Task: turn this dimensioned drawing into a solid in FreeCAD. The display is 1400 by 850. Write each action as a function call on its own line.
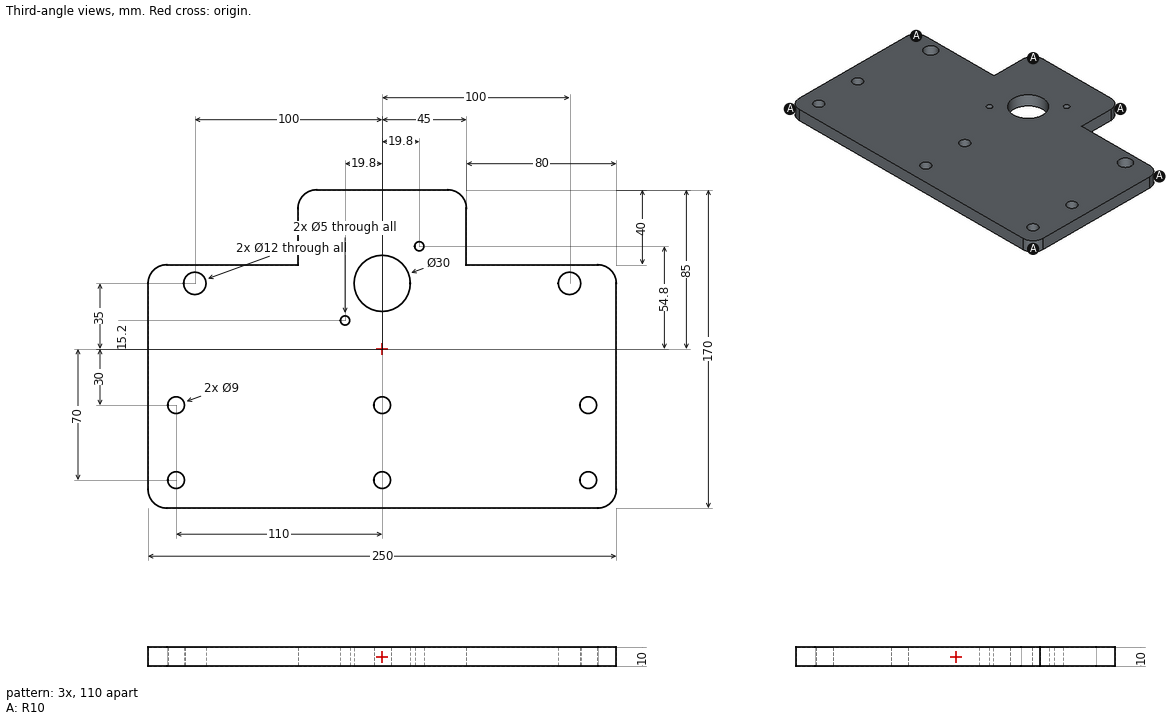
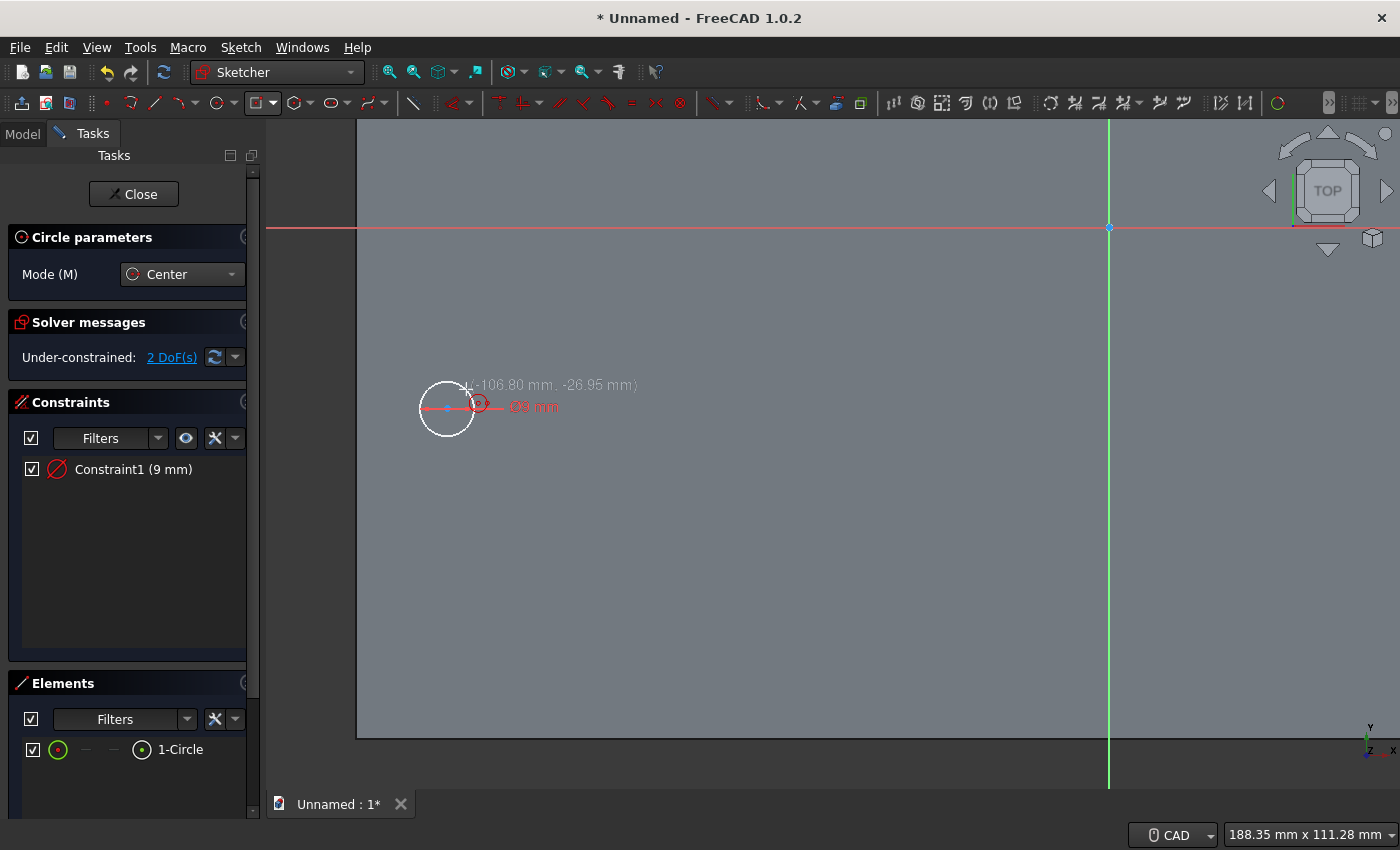
click(447, 649)
move(466, 630)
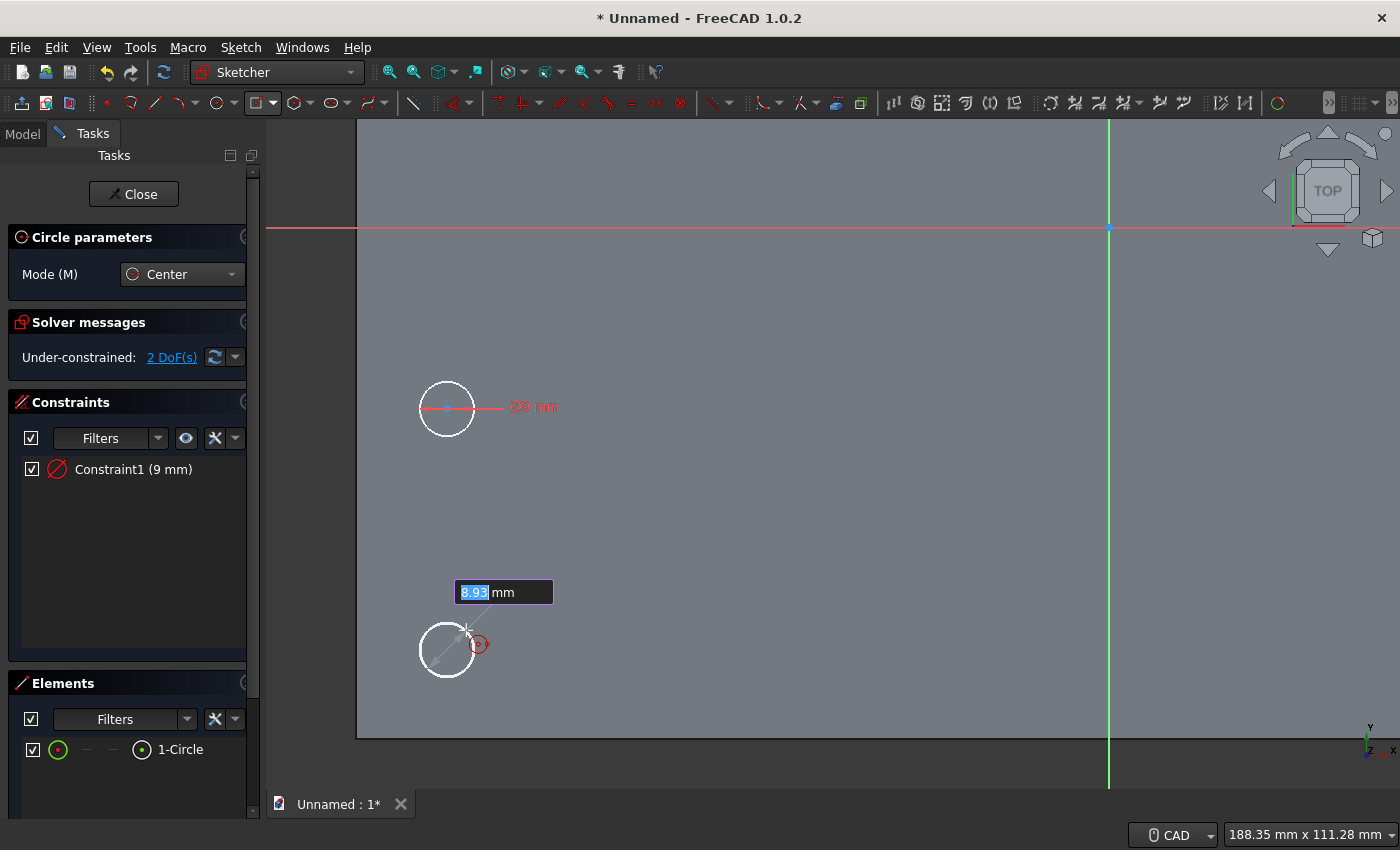
text(9)
key(Return)
key(Escape)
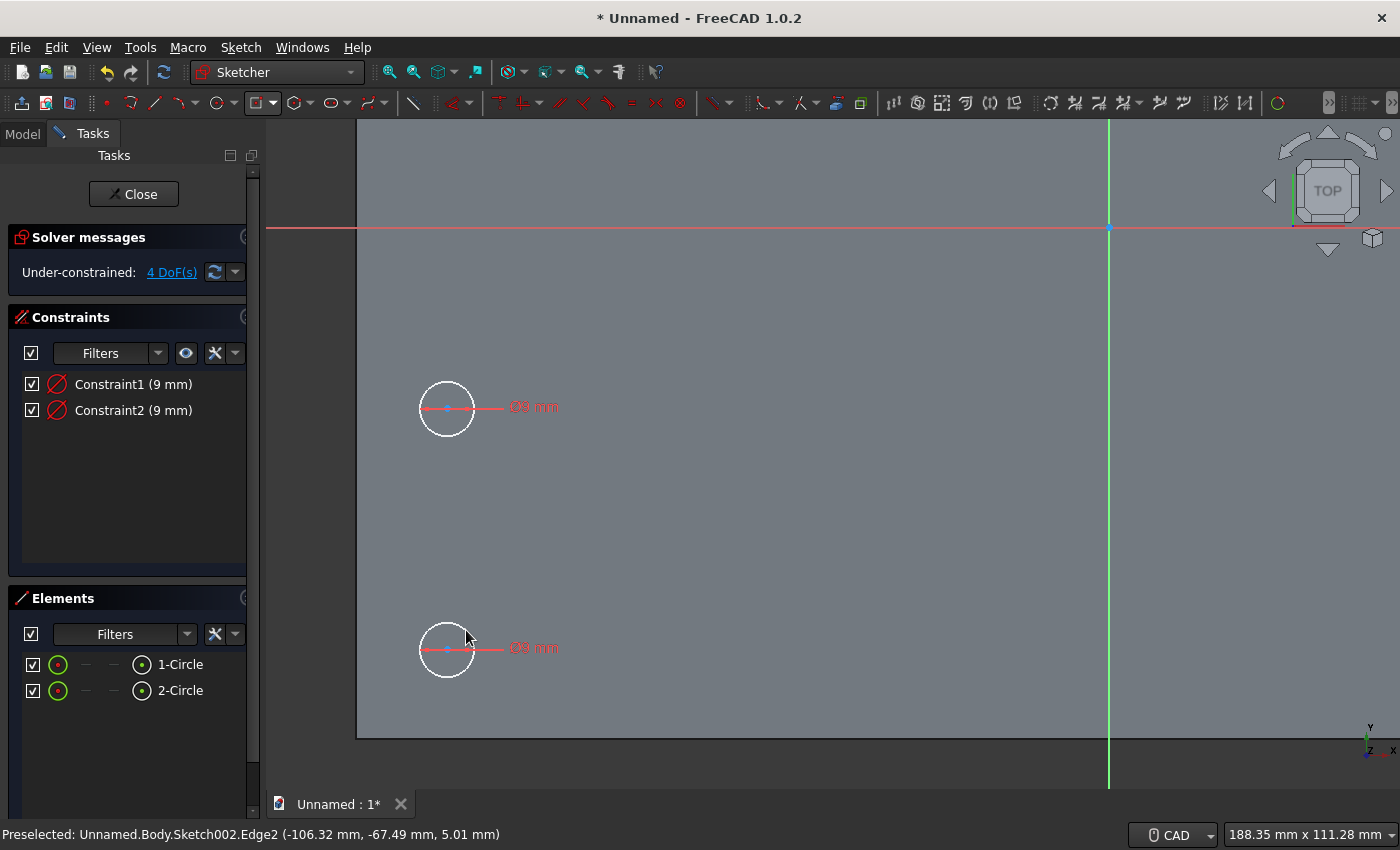
click(447, 409)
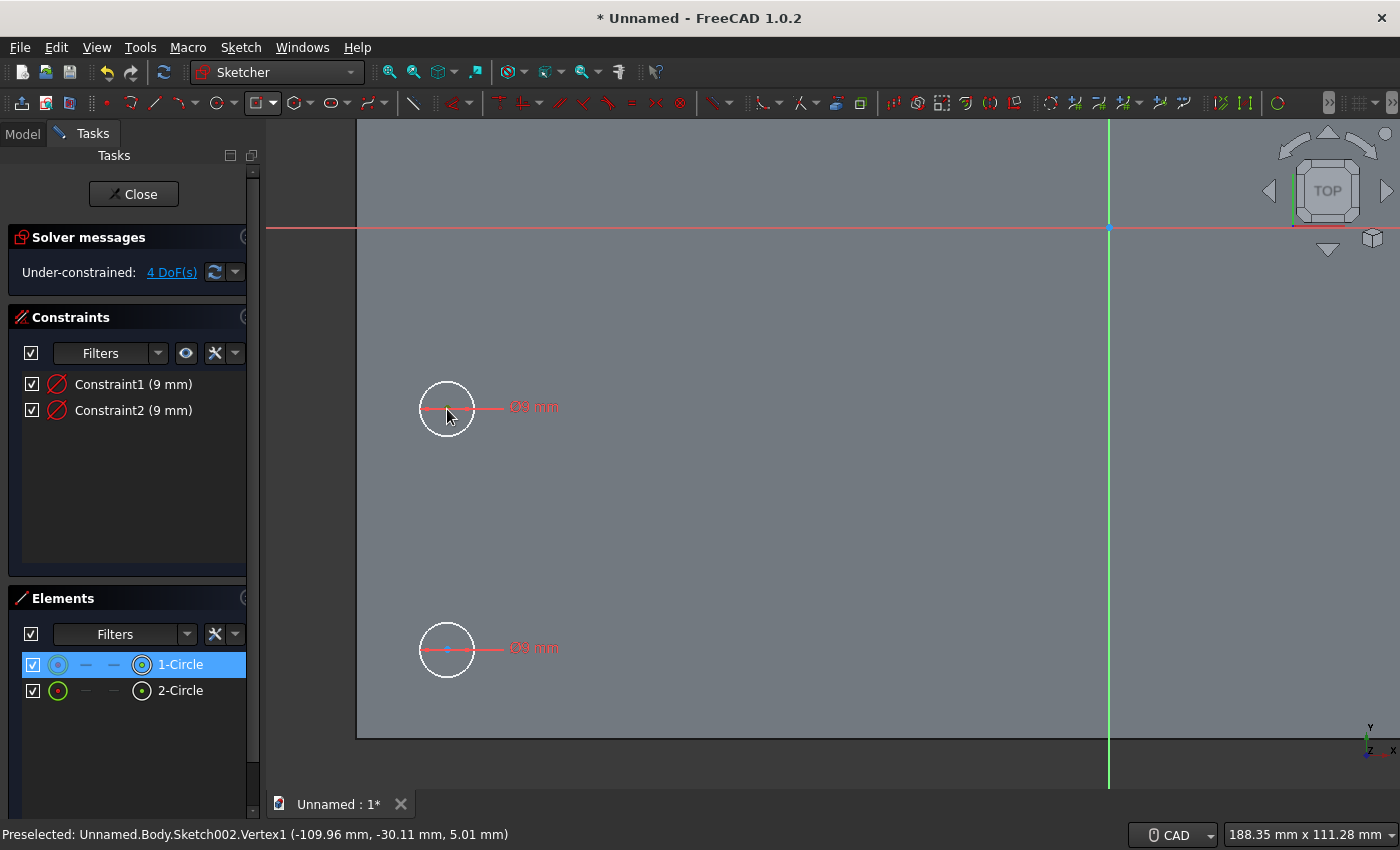
click(447, 650)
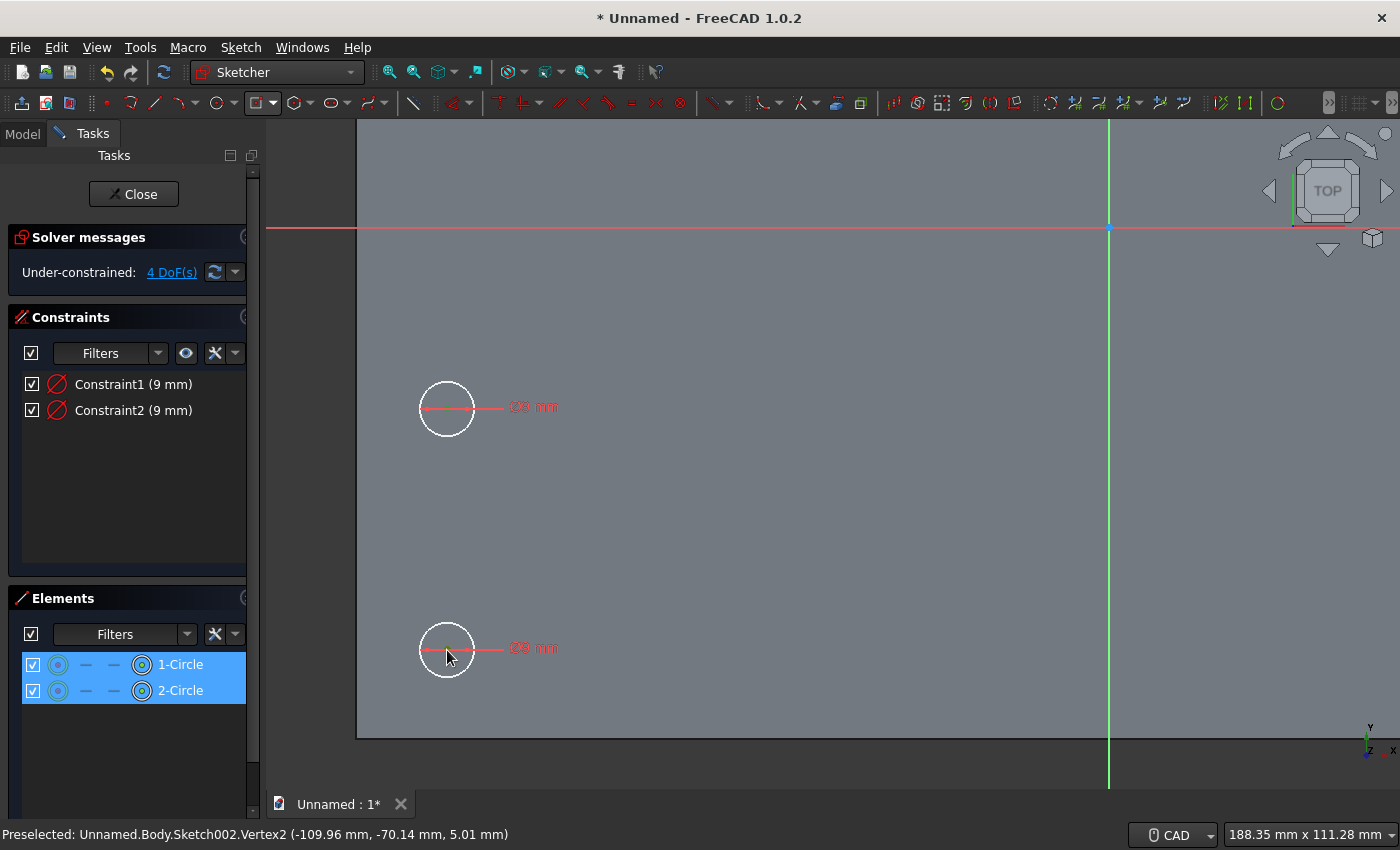
click(542, 104)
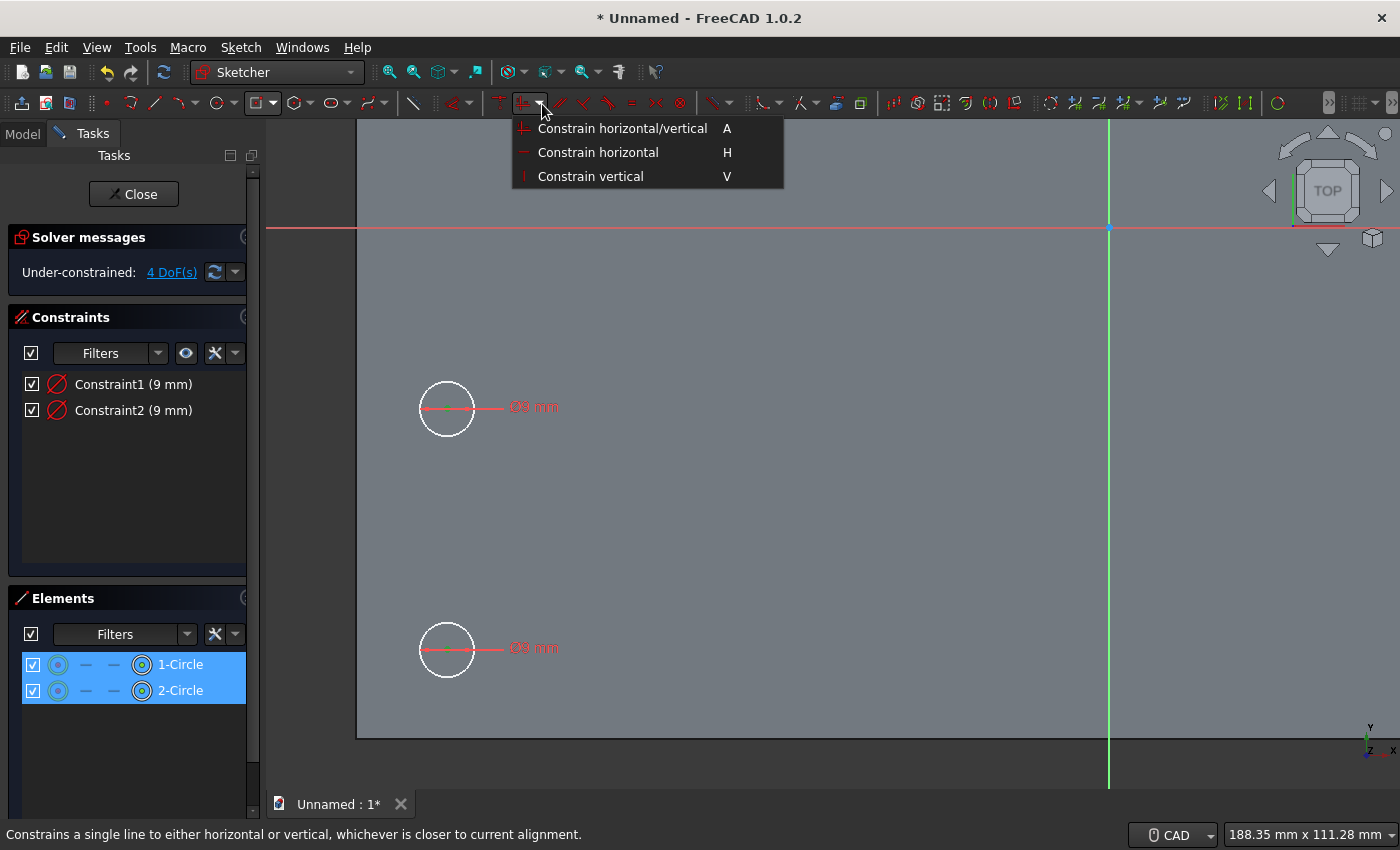
click(648, 176)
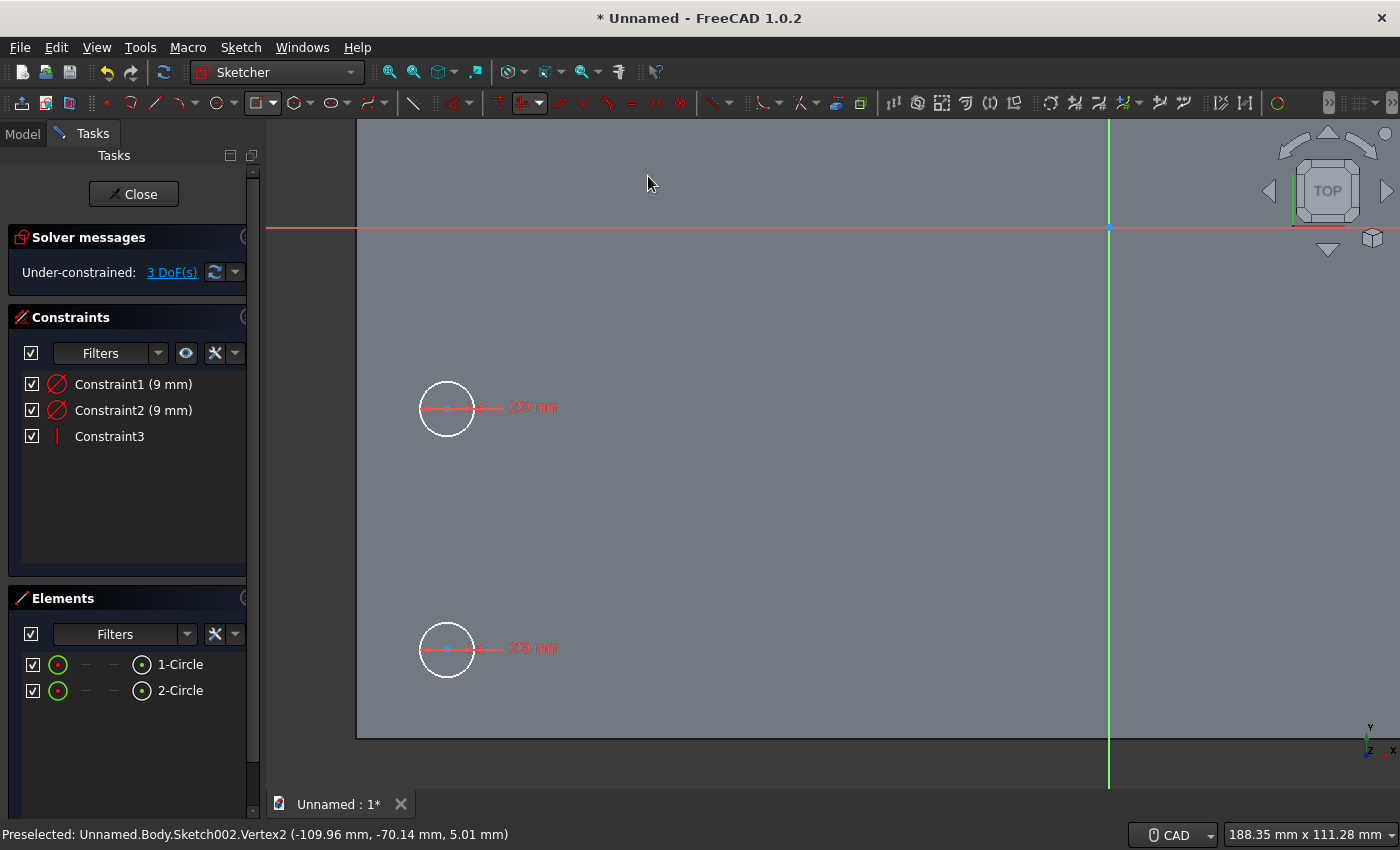
click(452, 104)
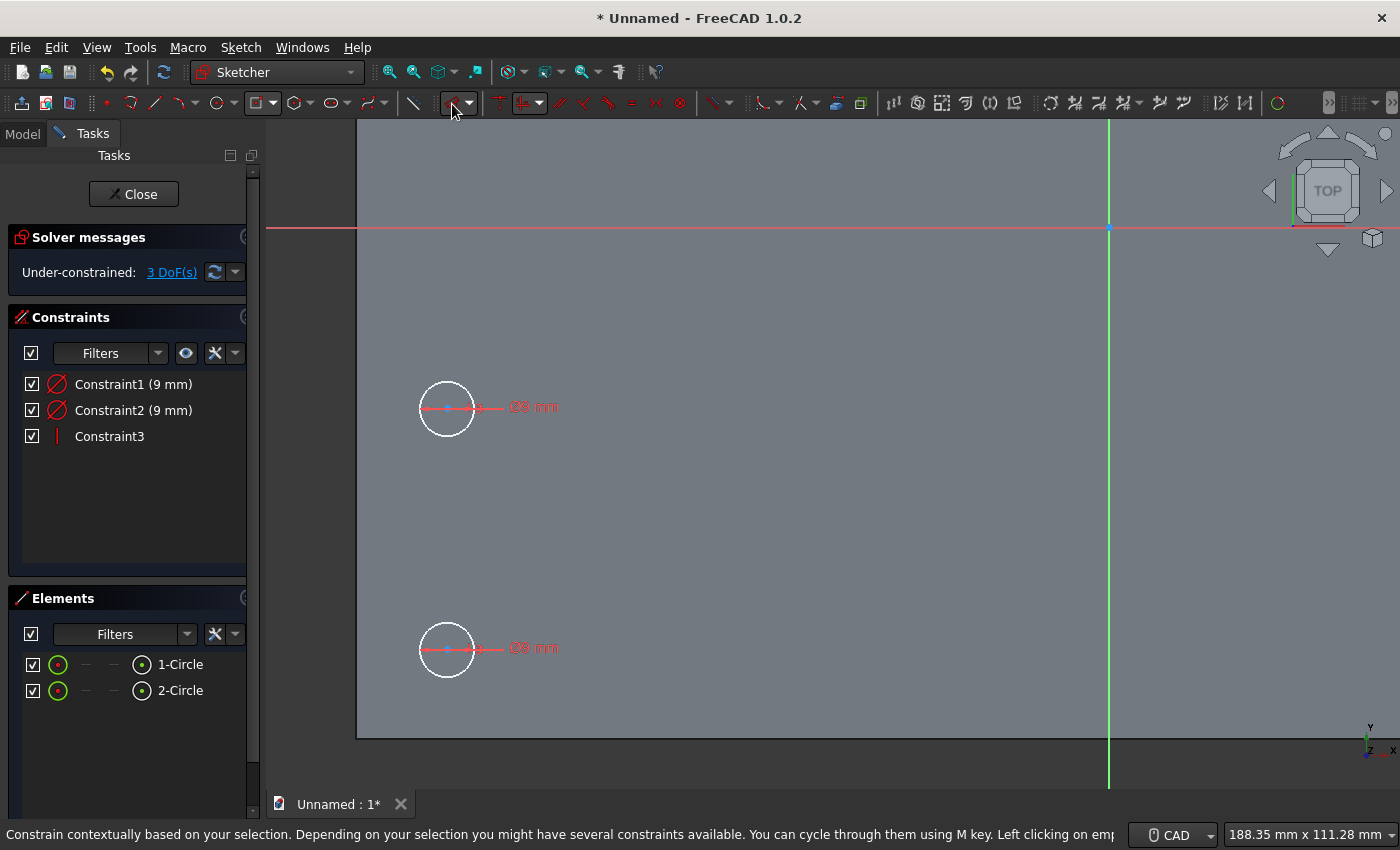
click(447, 409)
click(1143, 318)